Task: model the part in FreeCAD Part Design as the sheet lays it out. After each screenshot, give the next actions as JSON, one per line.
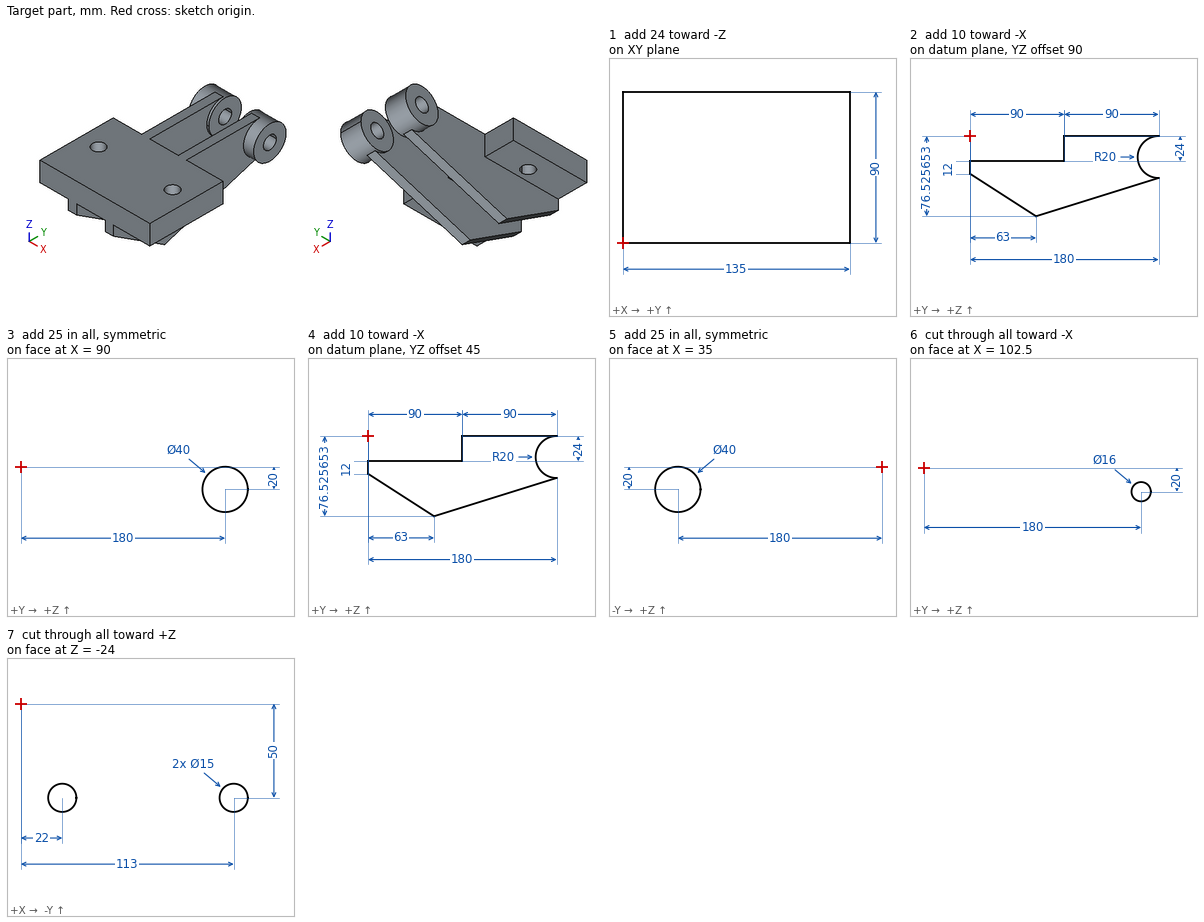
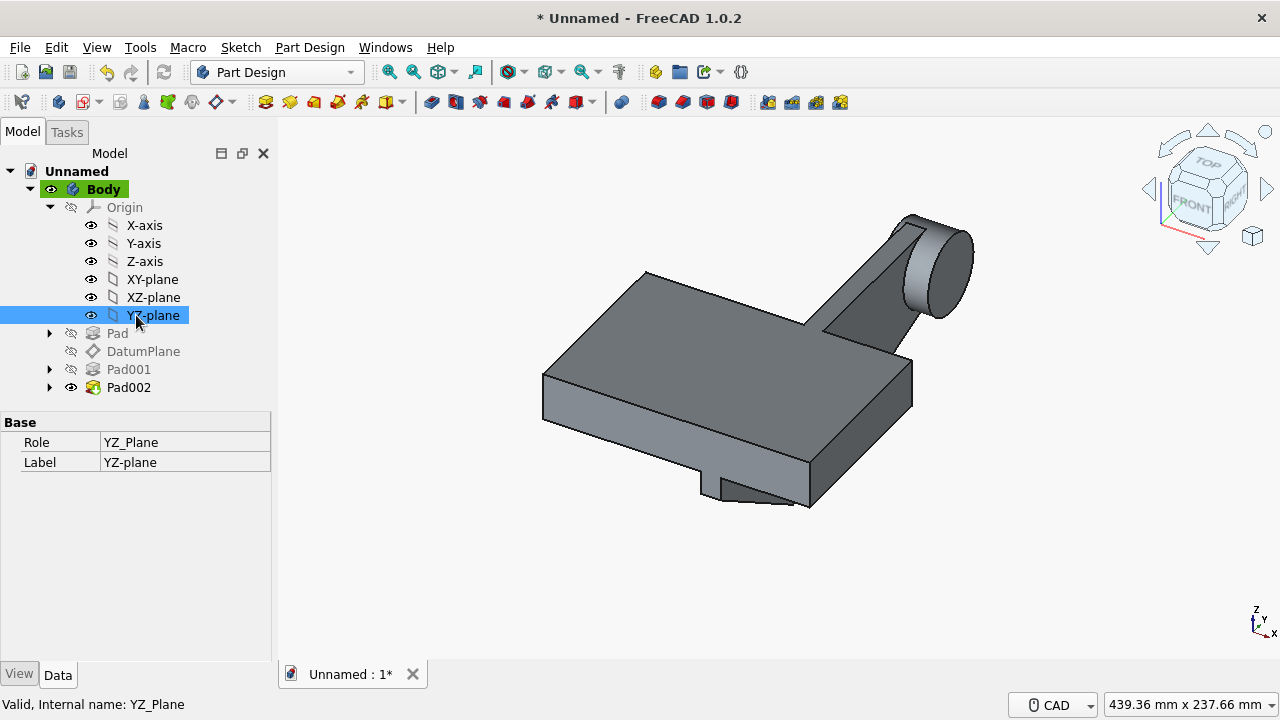
{"action": "left_click", "coordinate": [216, 102]}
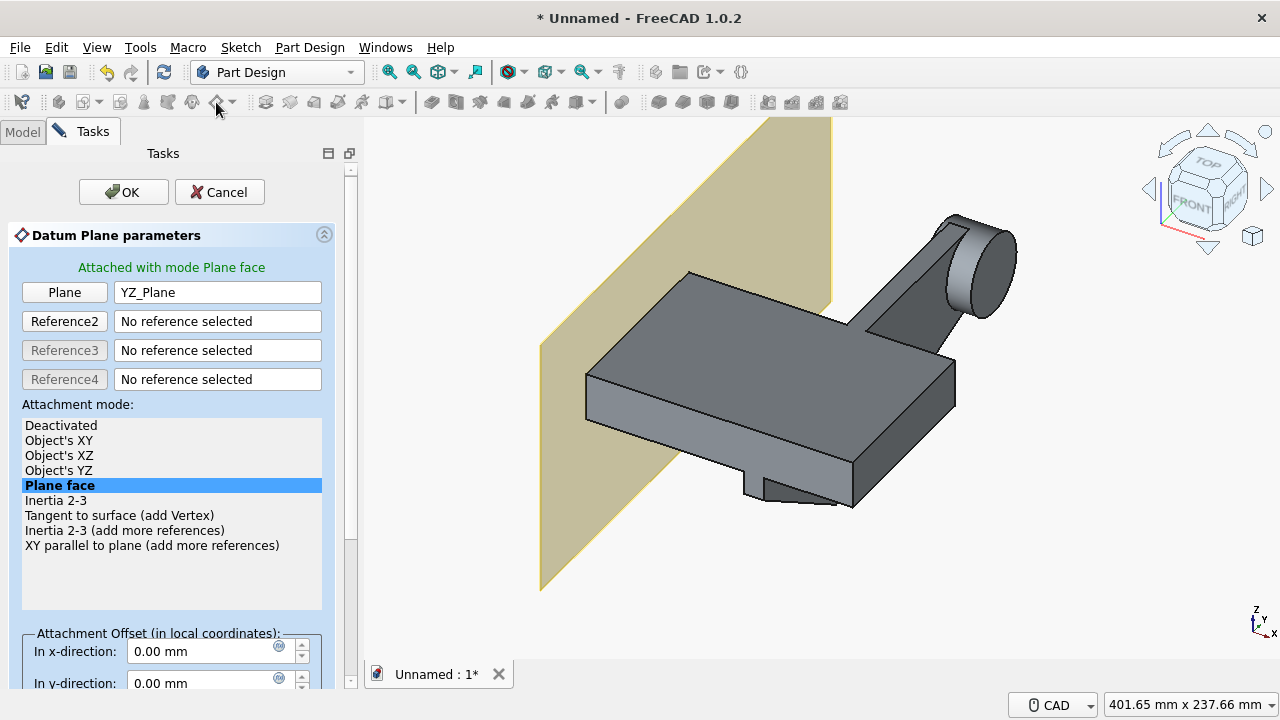
{"action": "scroll", "coordinate": [351, 426], "scroll_direction": "down", "scroll_amount": 2}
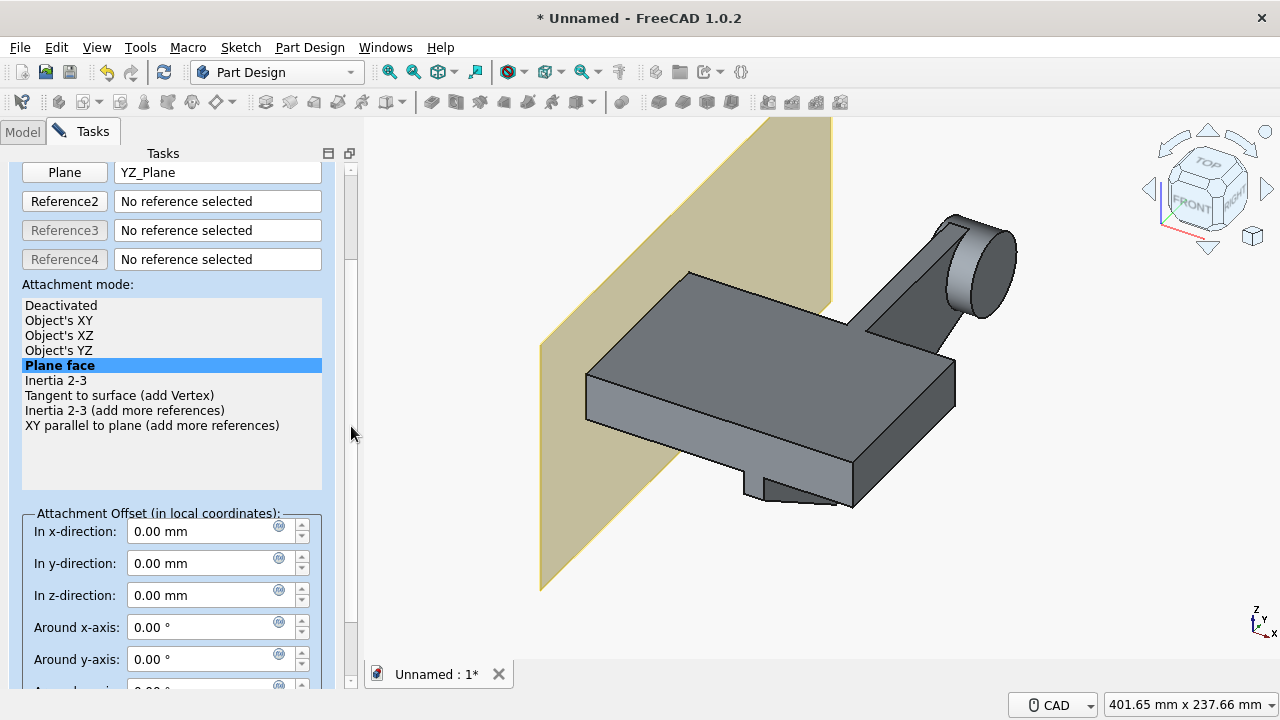
{"action": "triple_click", "coordinate": [210, 595]}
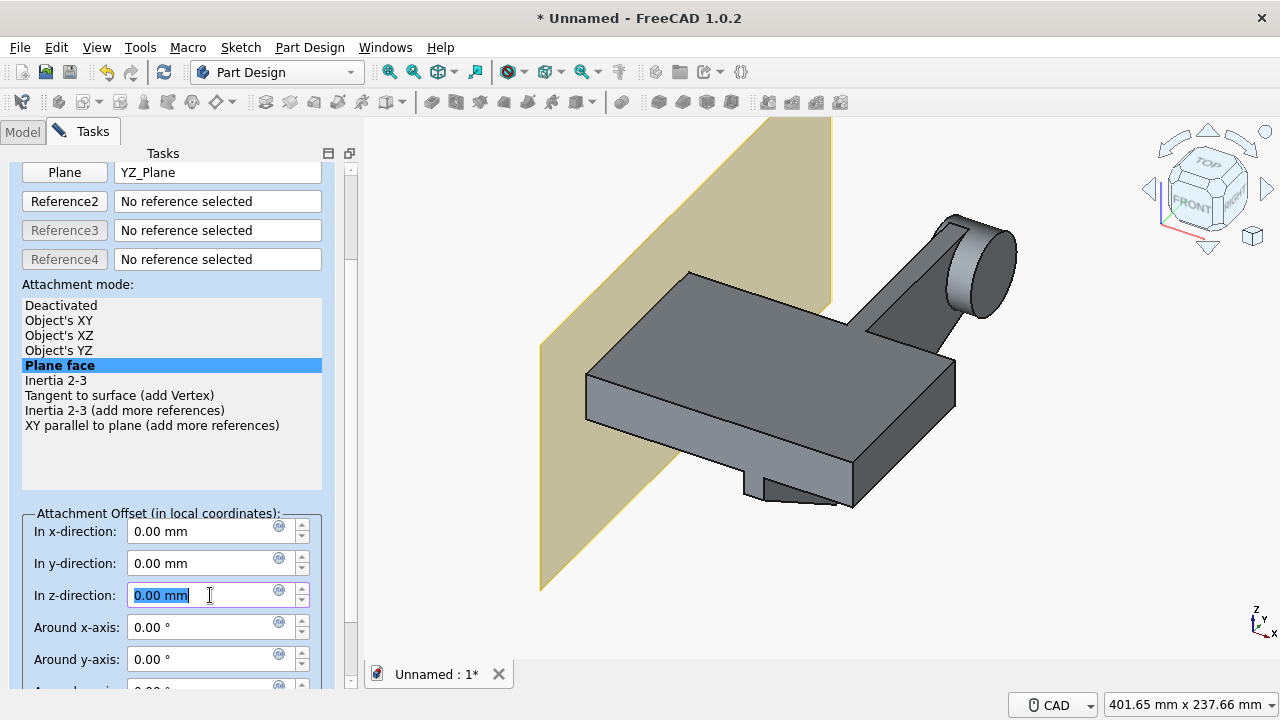
{"action": "type", "text": "45"}
{"action": "key", "text": "Tab"}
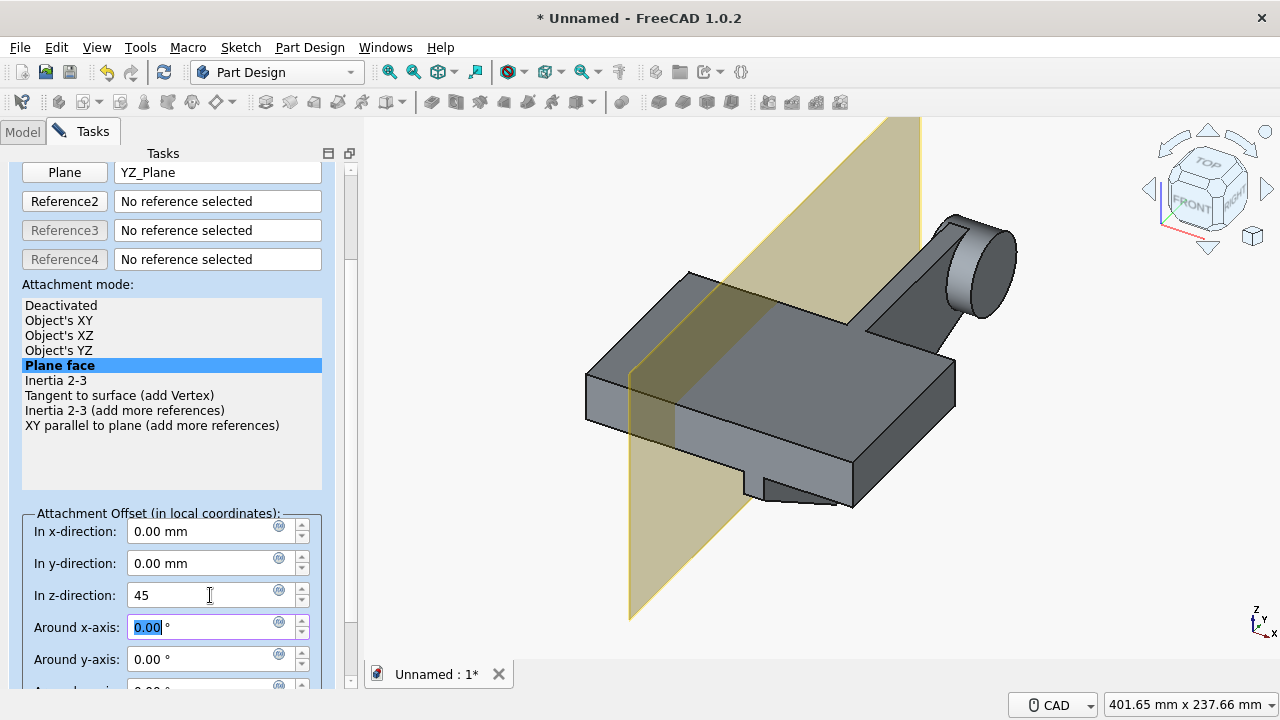
{"action": "scroll", "coordinate": [351, 426], "scroll_direction": "up", "scroll_amount": 3}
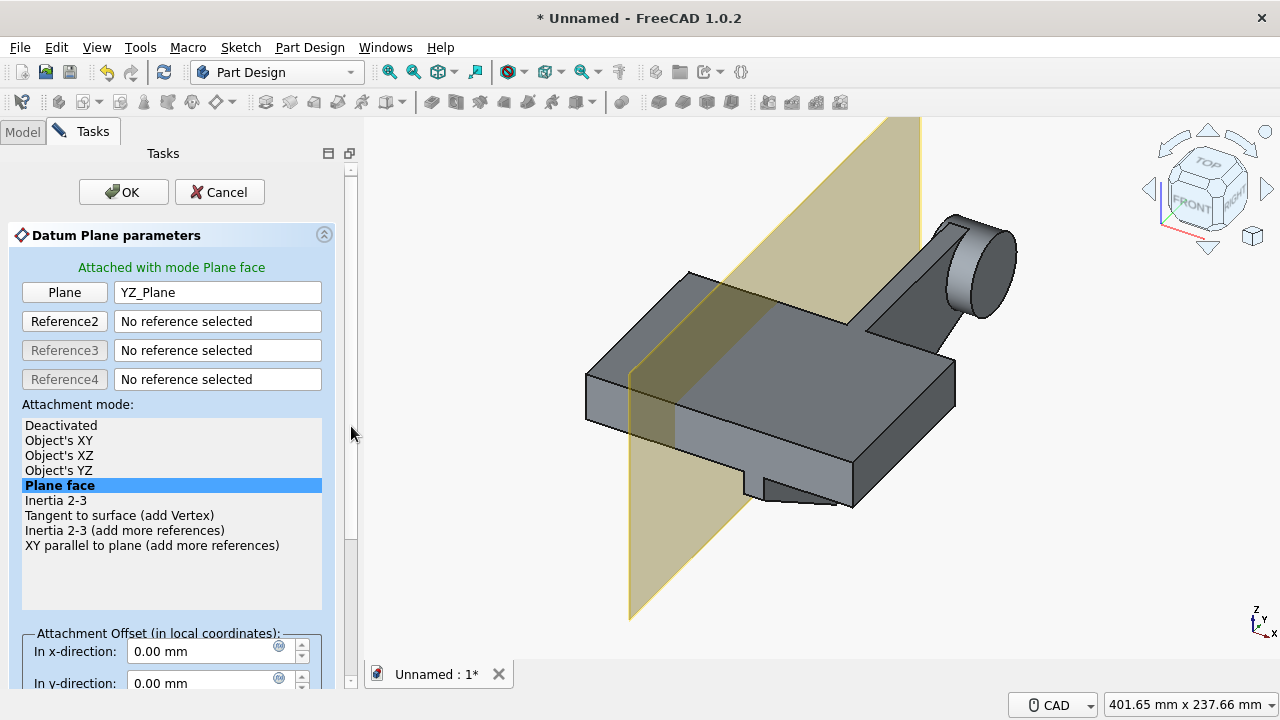
{"action": "left_click", "coordinate": [124, 192]}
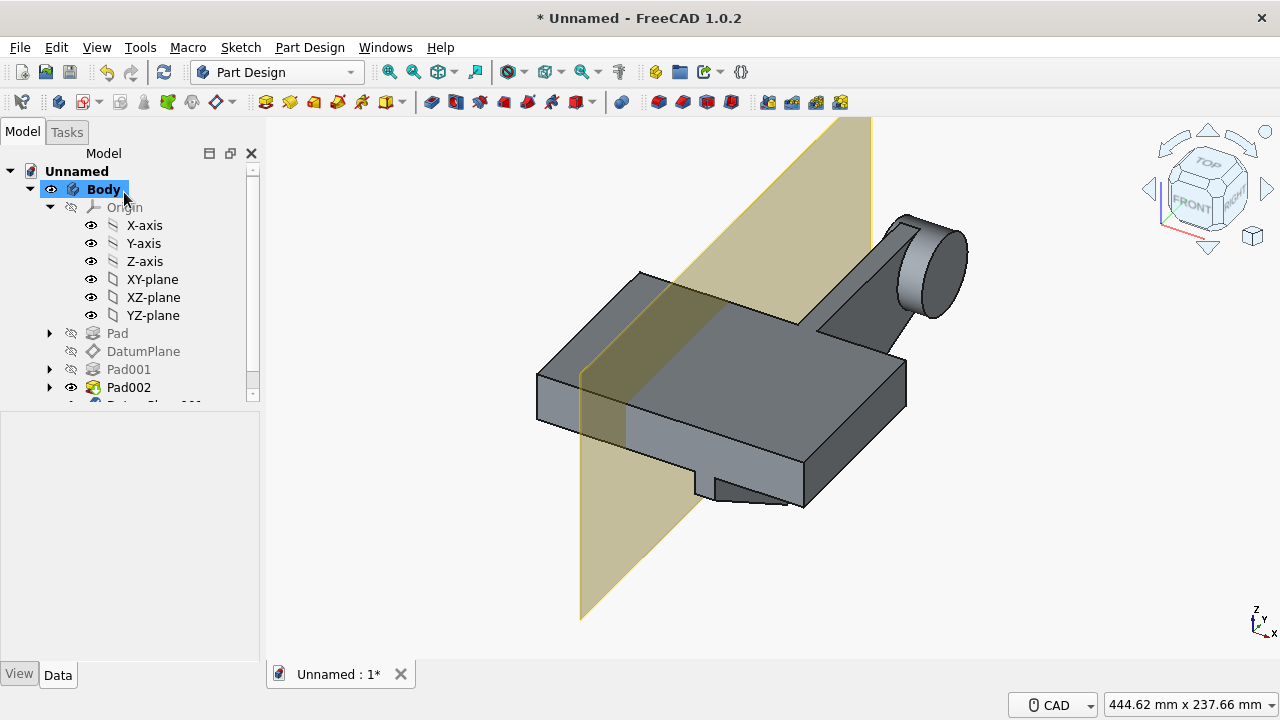
{"action": "scroll", "coordinate": [100, 275], "scroll_direction": "down", "scroll_amount": 3}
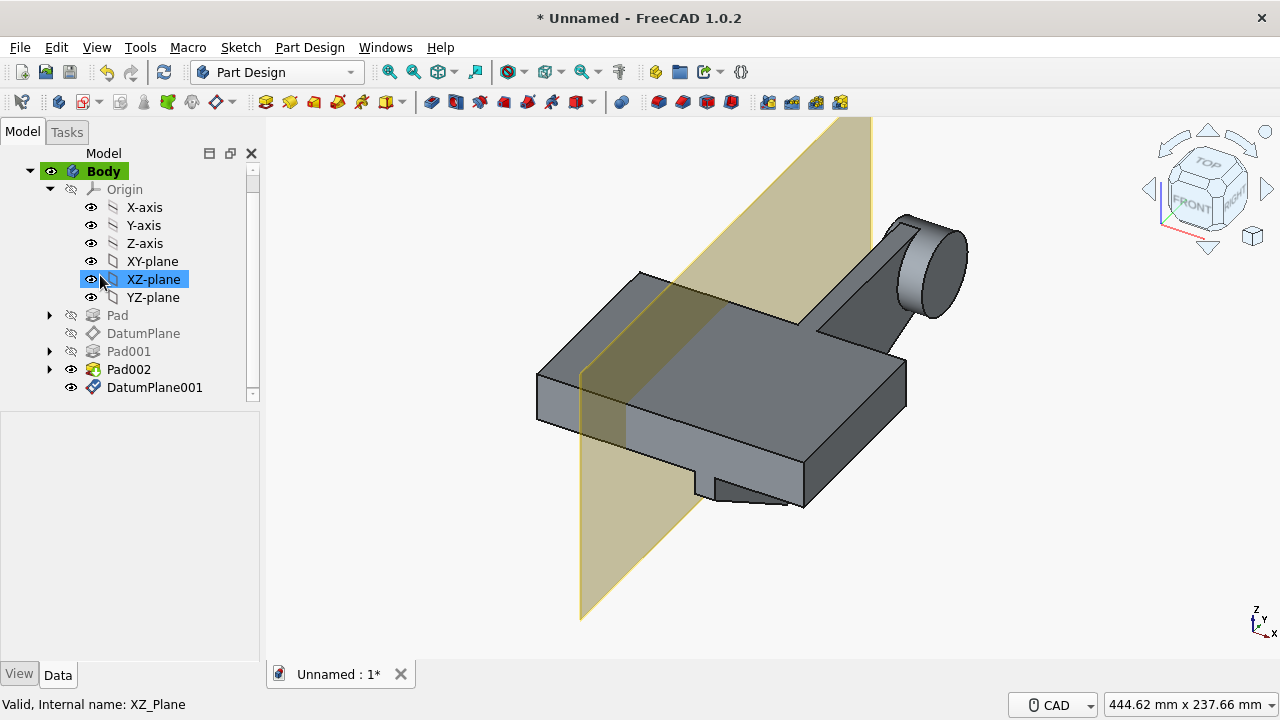
{"action": "left_click", "coordinate": [116, 387]}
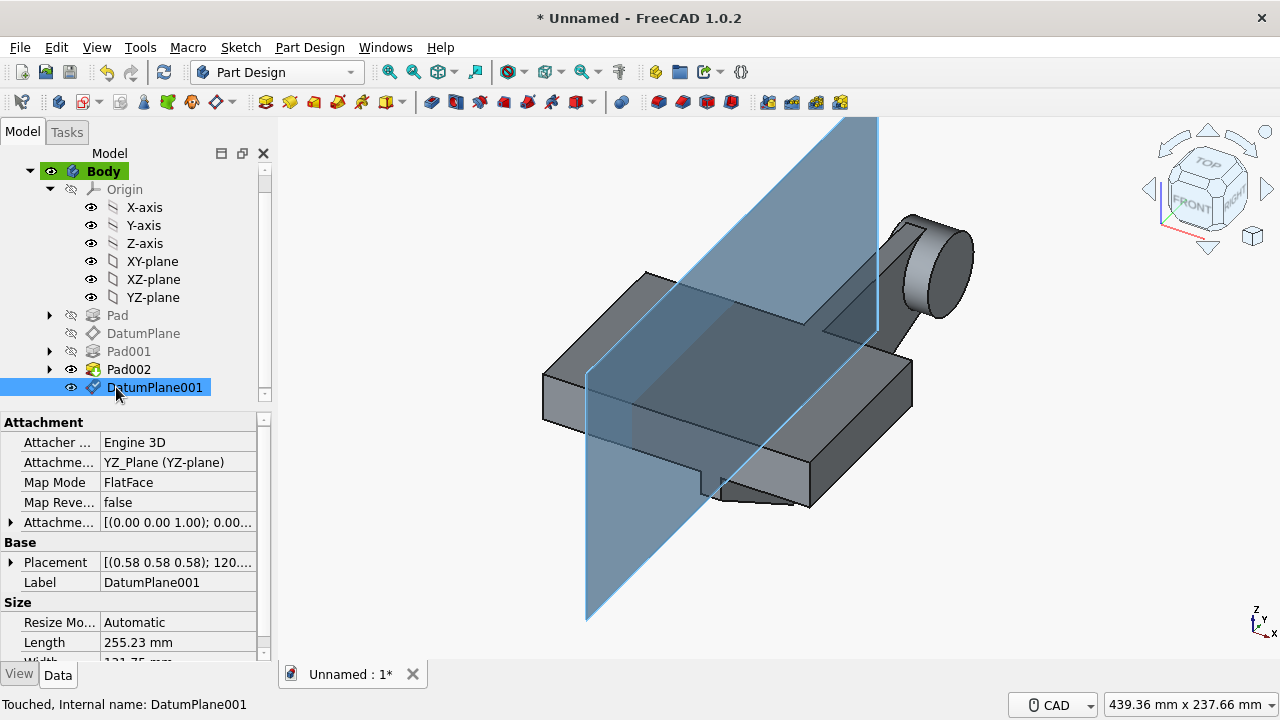
{"action": "left_click", "coordinate": [84, 102]}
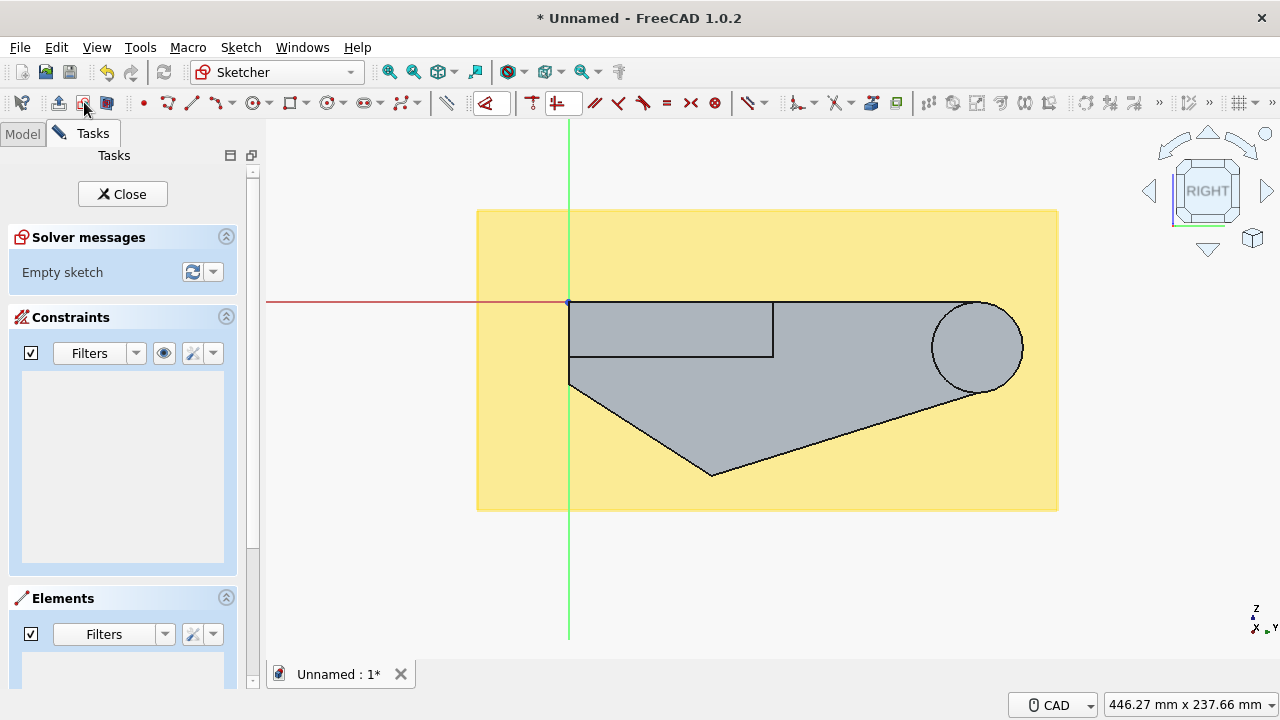
{"action": "left_click", "coordinate": [108, 104]}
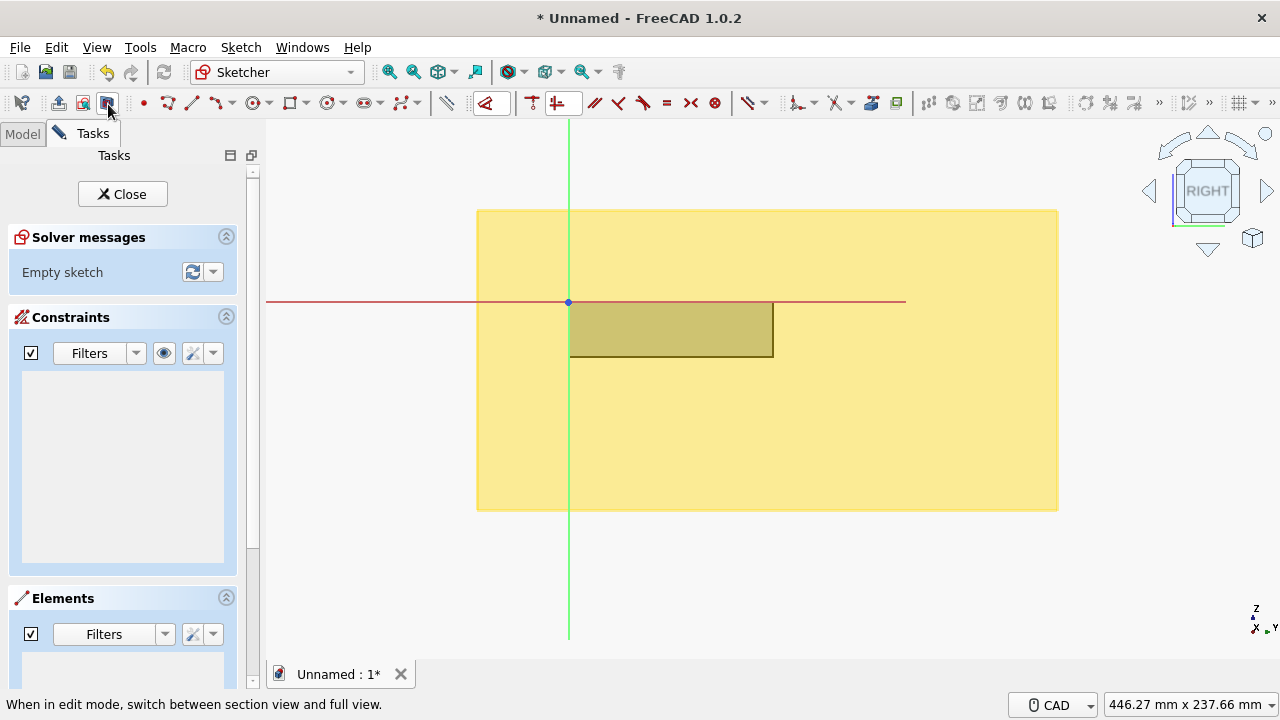
{"action": "scroll", "coordinate": [912, 389], "scroll_direction": "up", "scroll_amount": 2}